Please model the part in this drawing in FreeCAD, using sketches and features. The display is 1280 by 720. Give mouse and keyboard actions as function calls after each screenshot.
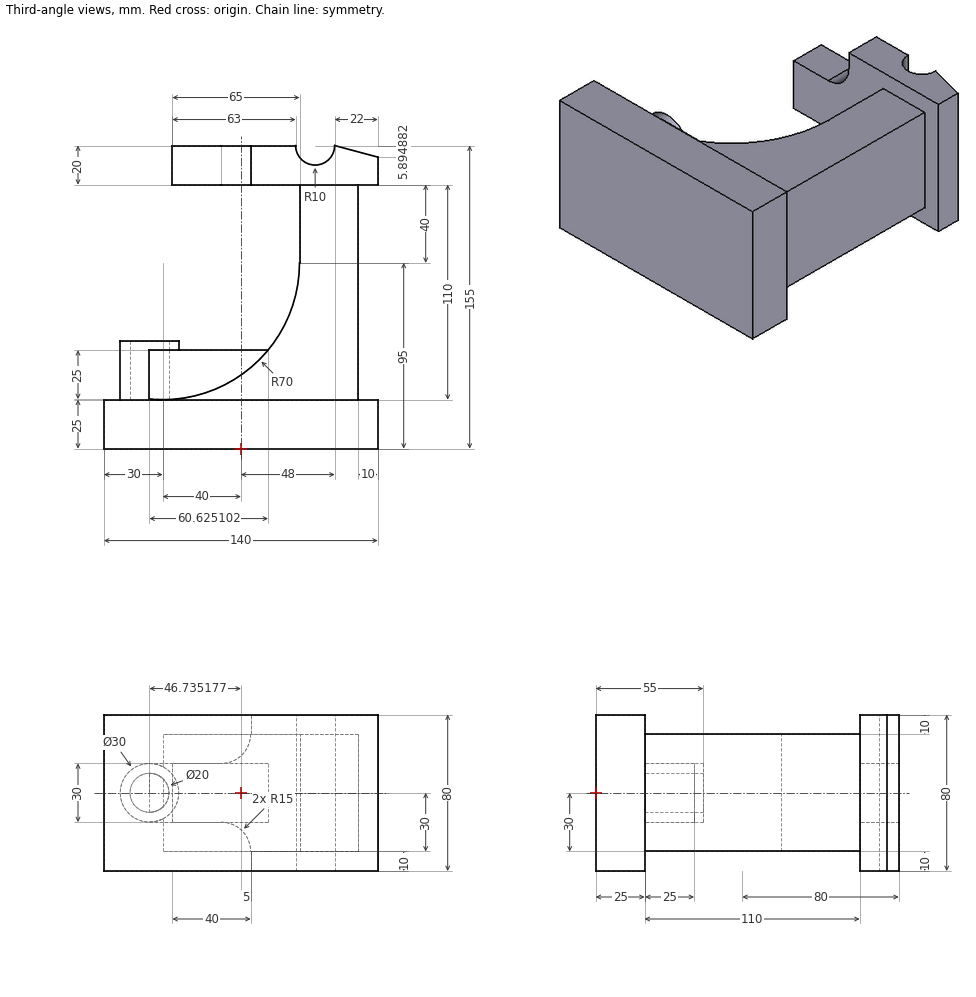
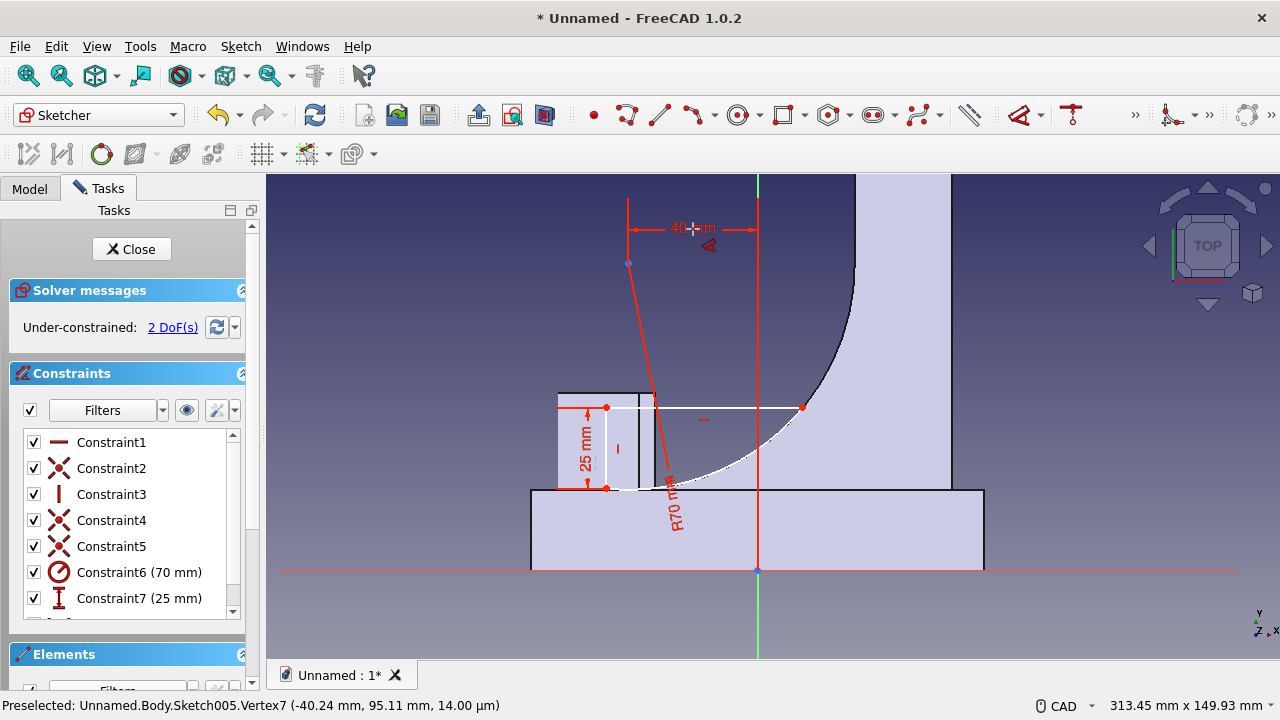
click(628, 263)
click(594, 346)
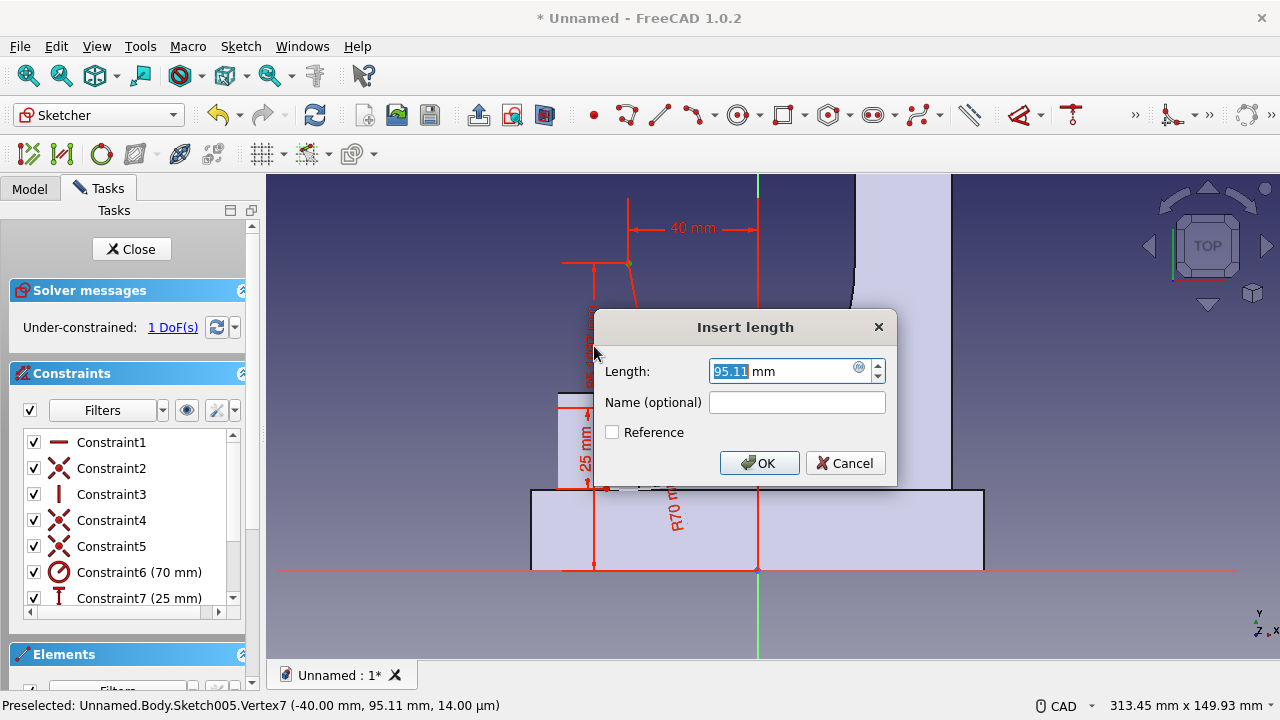
text(95)
key(Return)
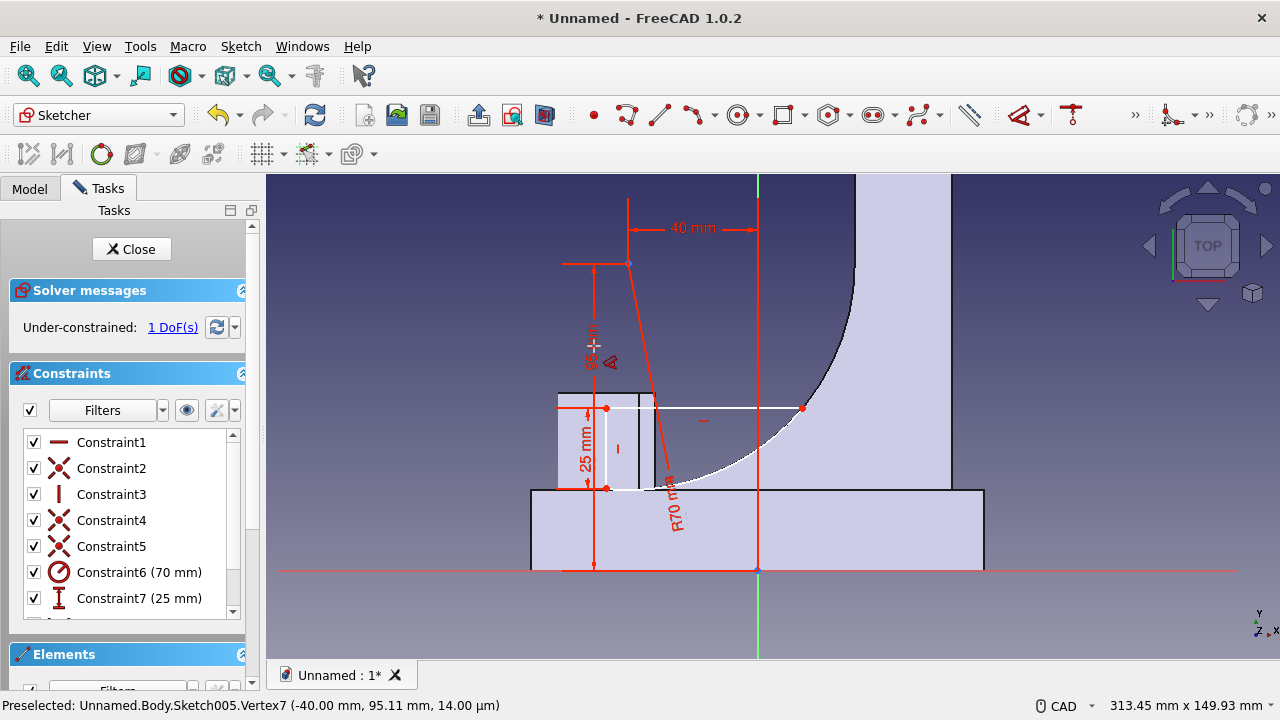
click(744, 408)
click(704, 374)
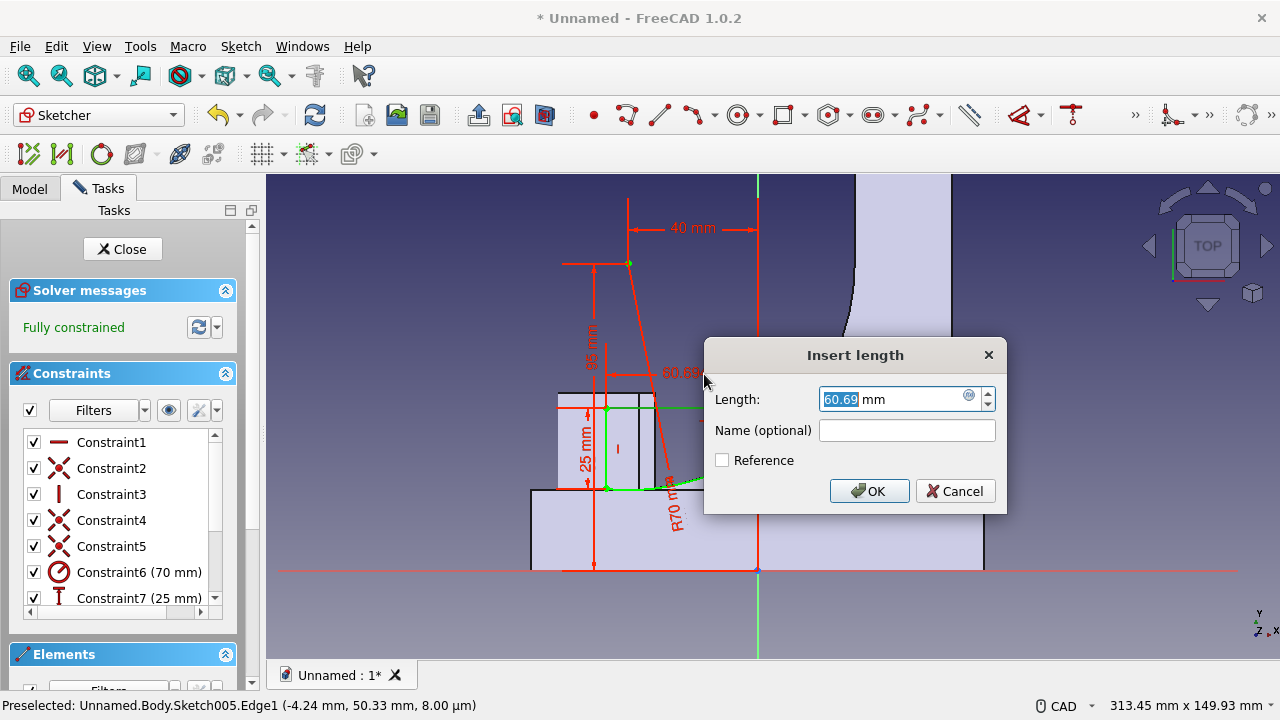
text(60.625102)
key(Return)
key(Escape)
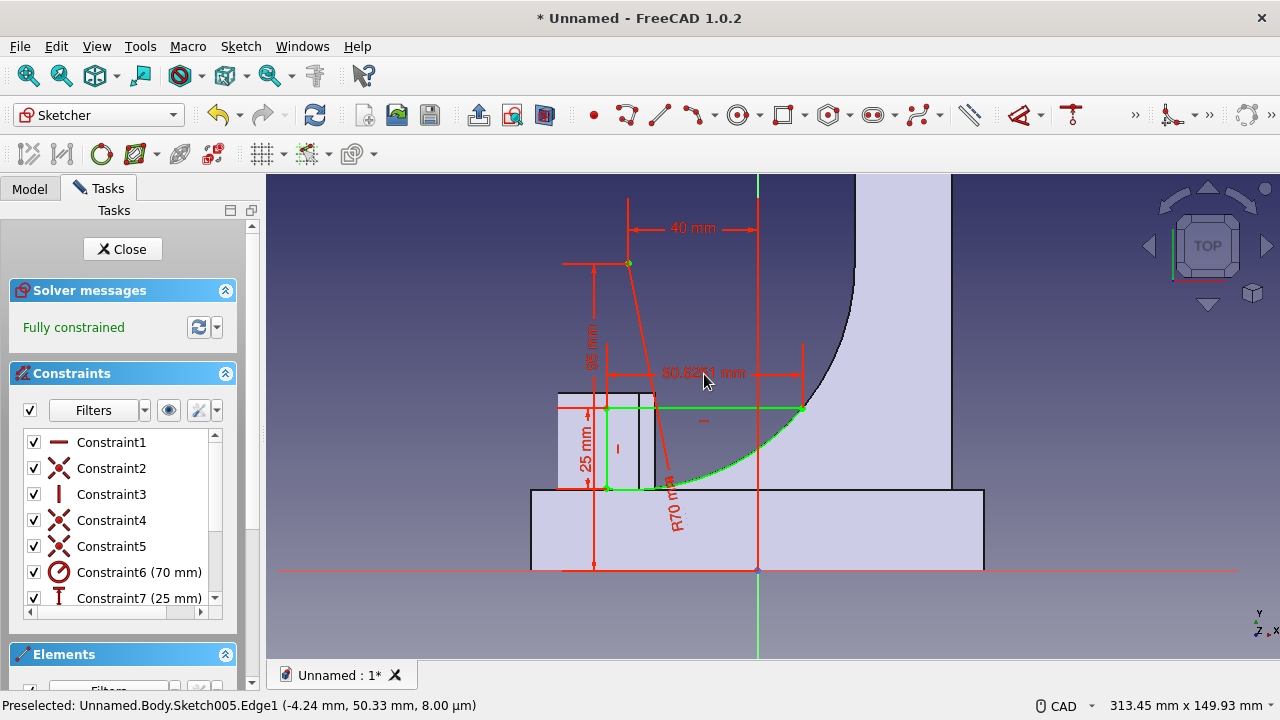
click(123, 249)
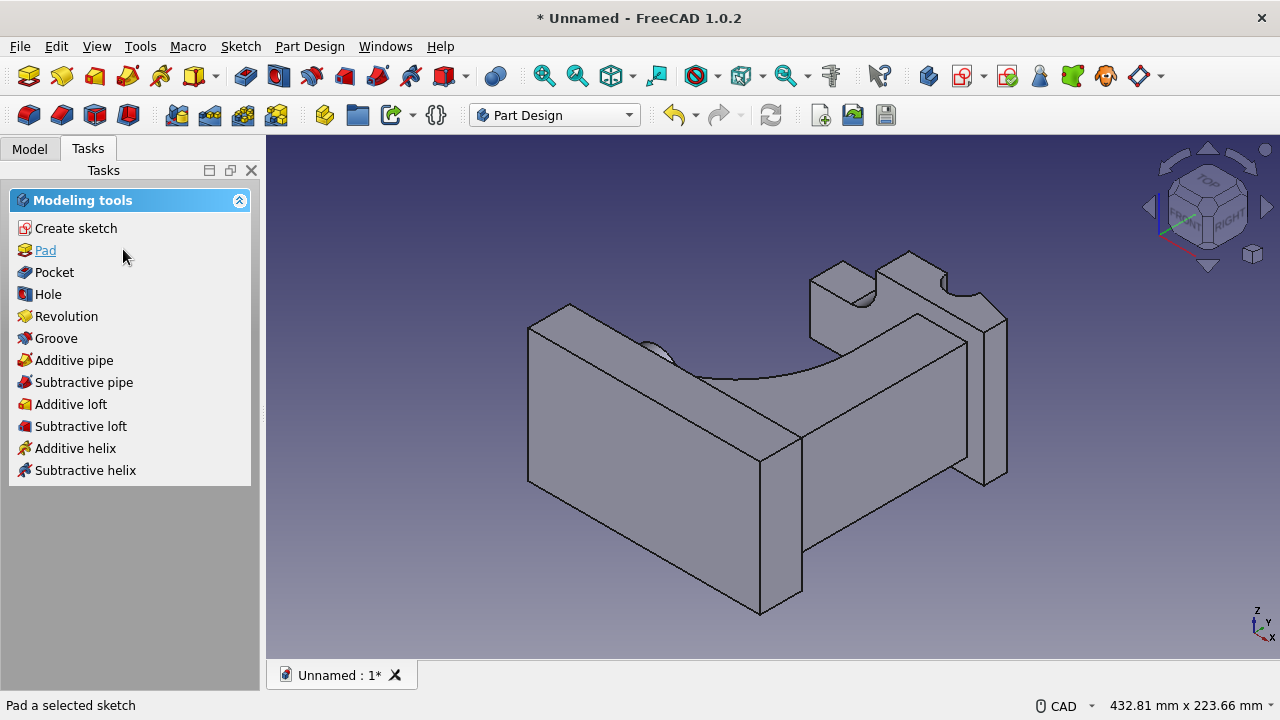
click(29, 76)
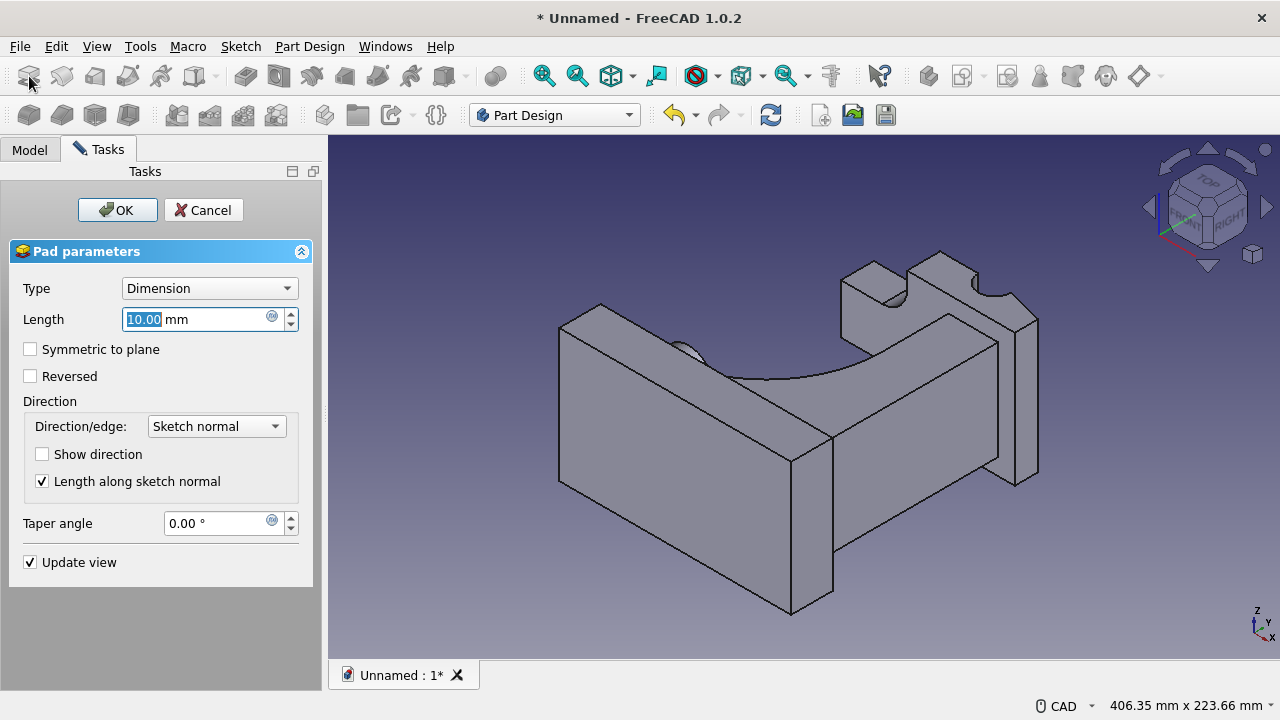
text(30)
key(Tab)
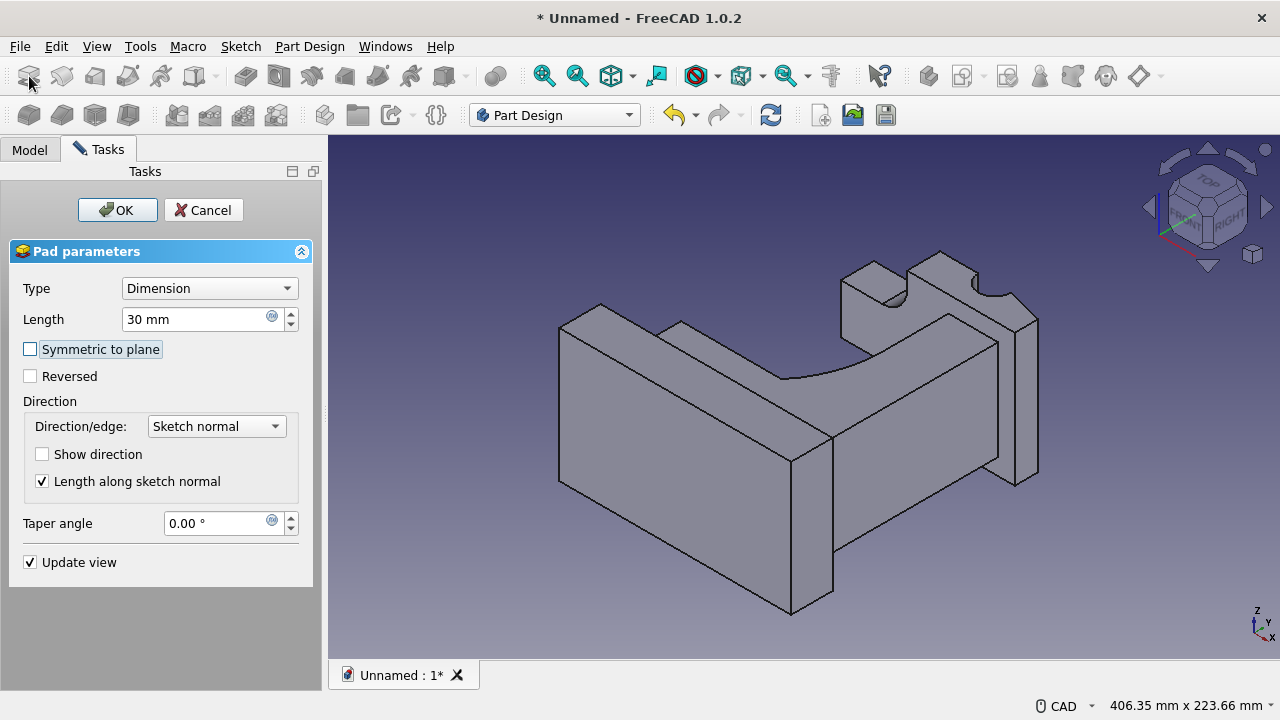
click(31, 349)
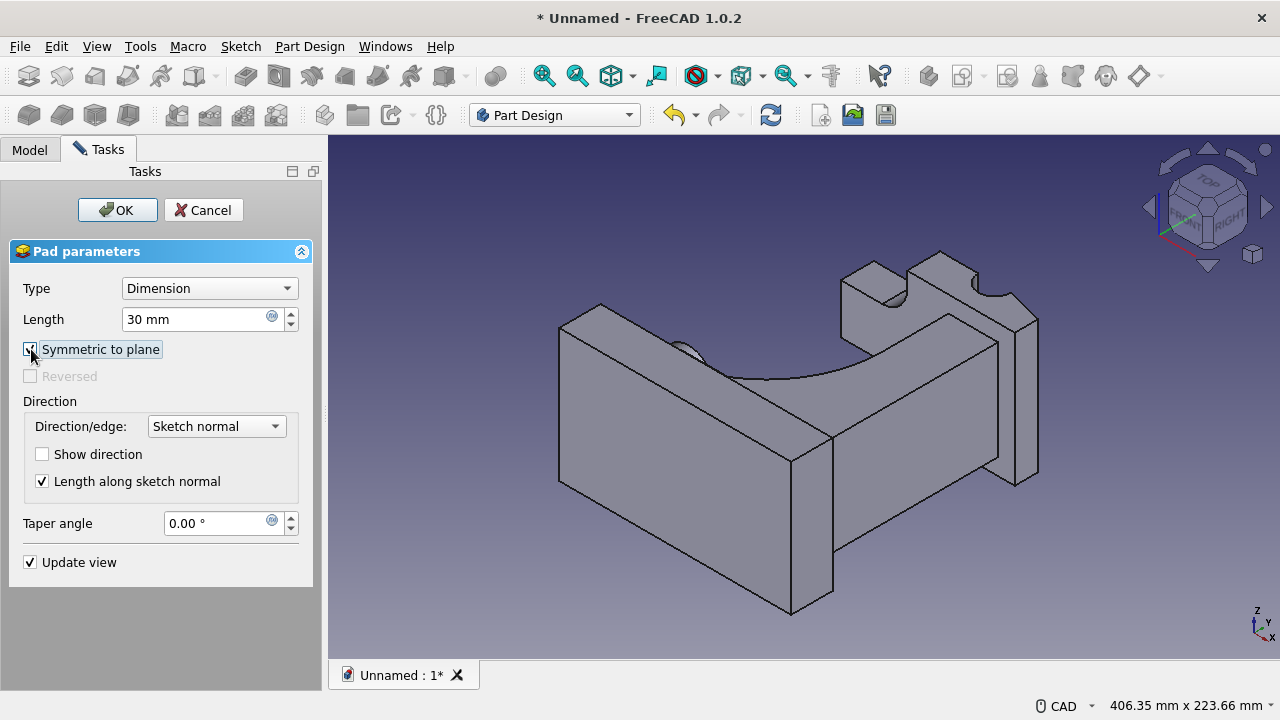
click(118, 210)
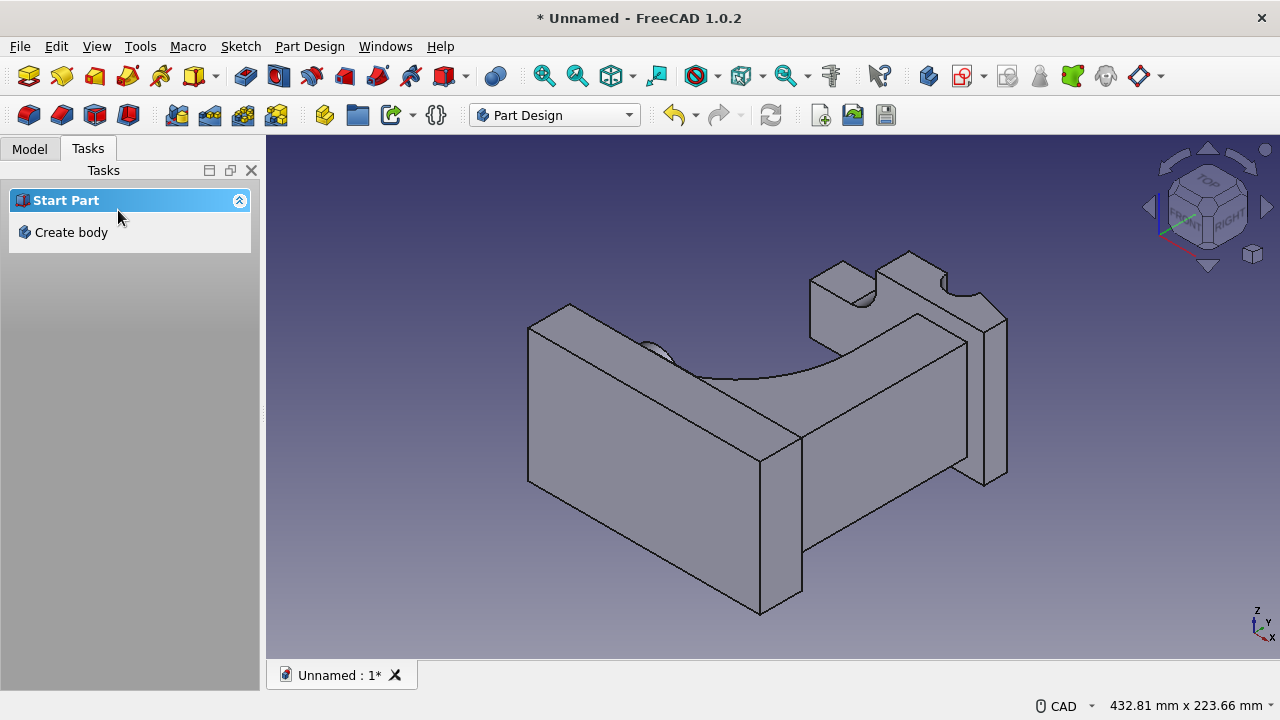
click(30, 148)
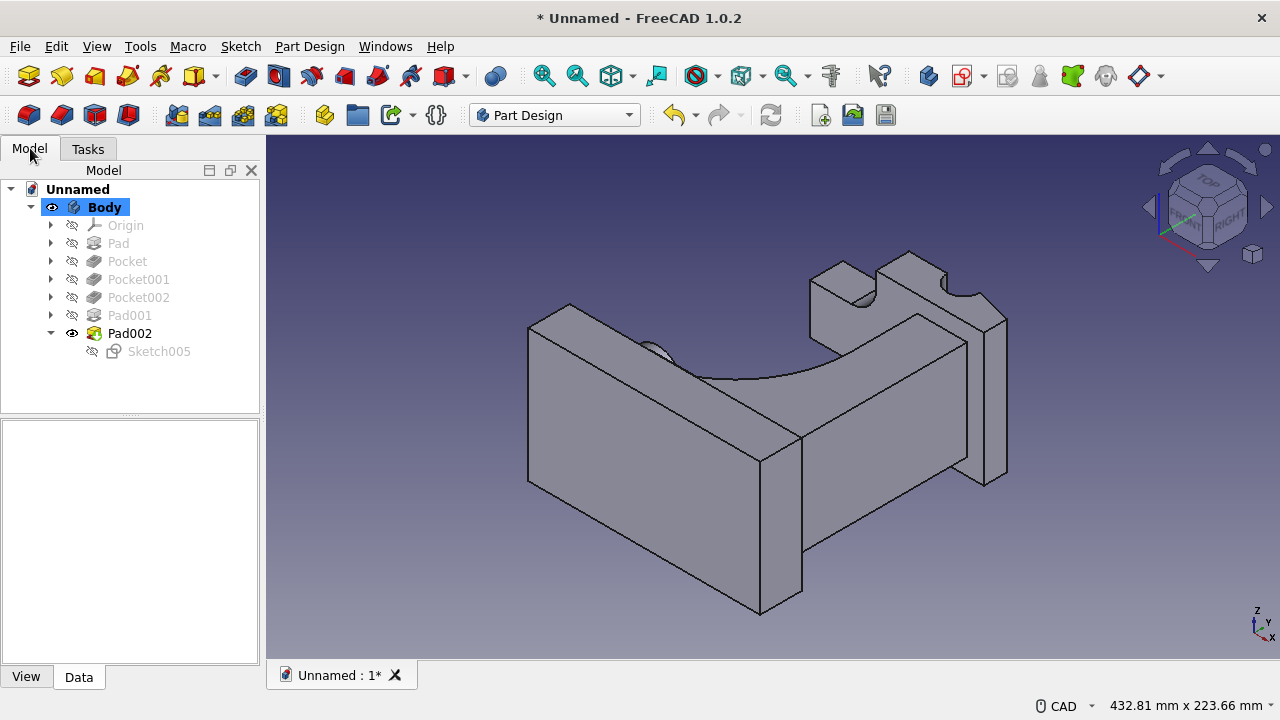
click(51, 225)